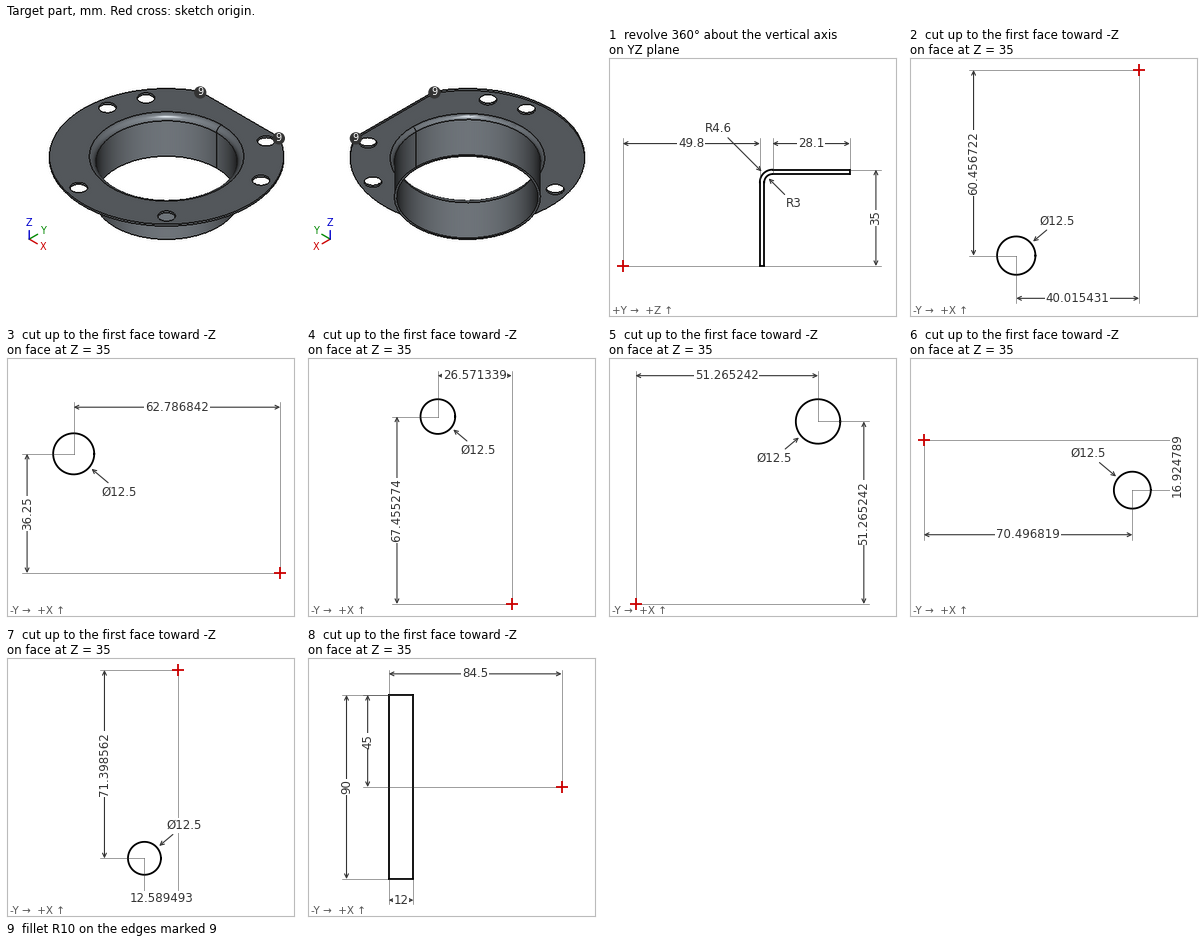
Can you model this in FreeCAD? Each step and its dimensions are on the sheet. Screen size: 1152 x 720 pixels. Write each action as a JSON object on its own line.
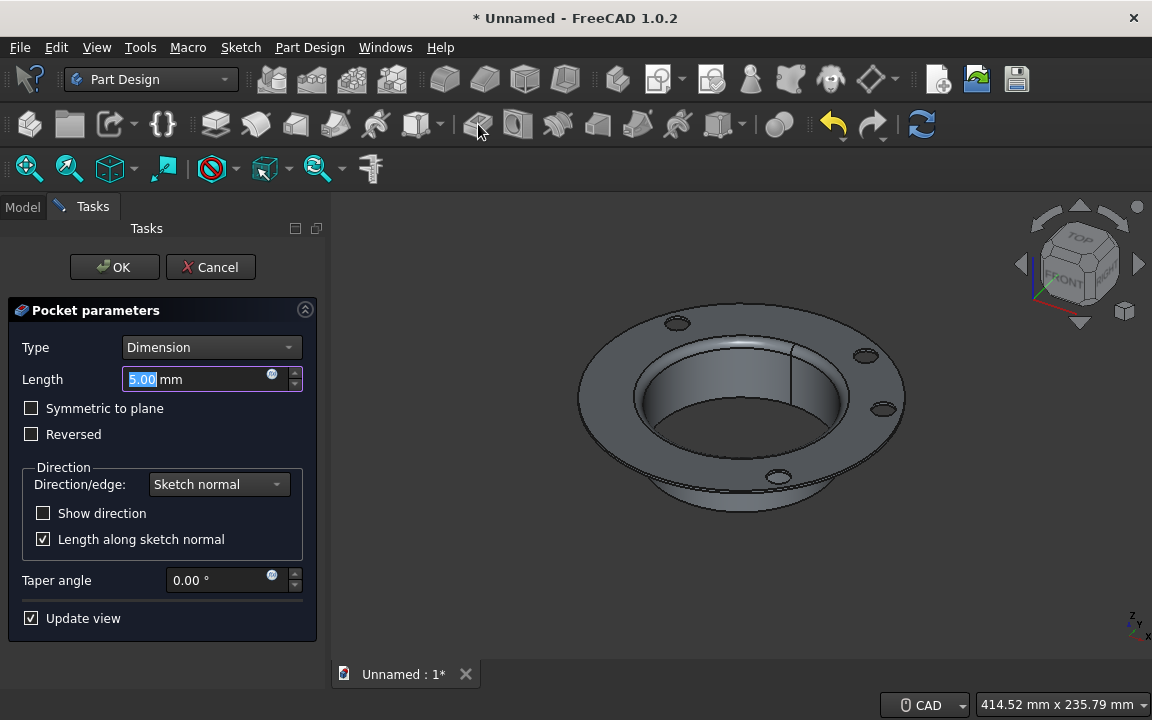
{"action": "left_click", "coordinate": [212, 348]}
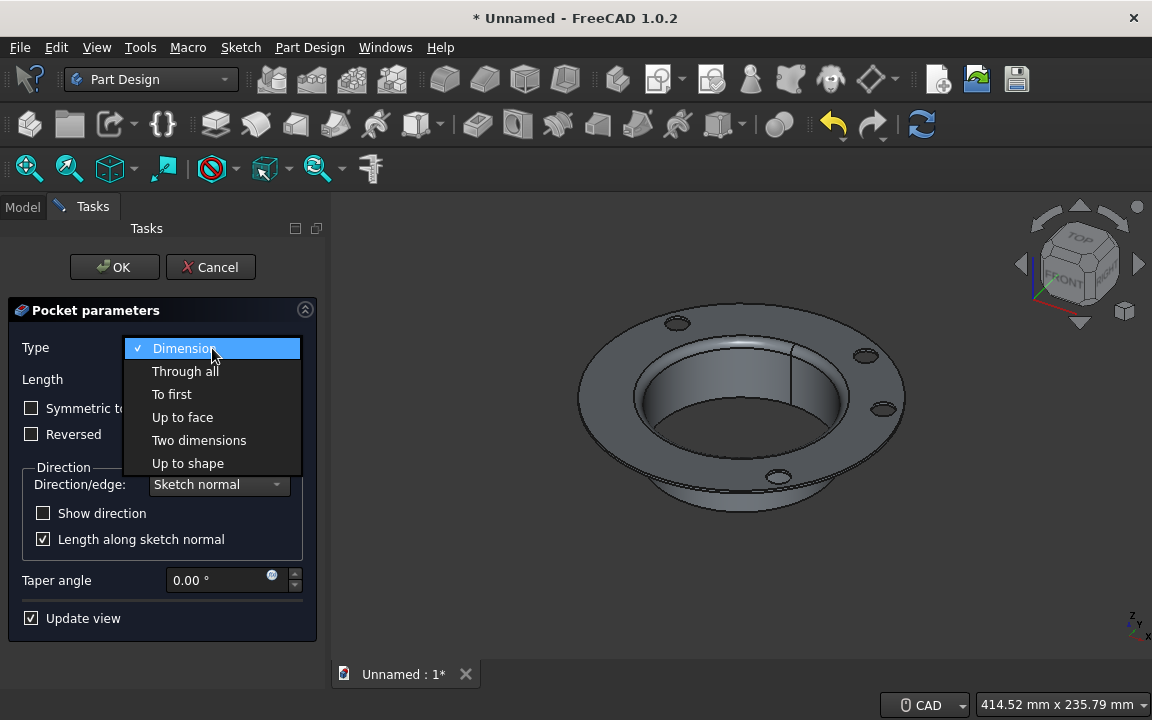
{"action": "left_click", "coordinate": [212, 394]}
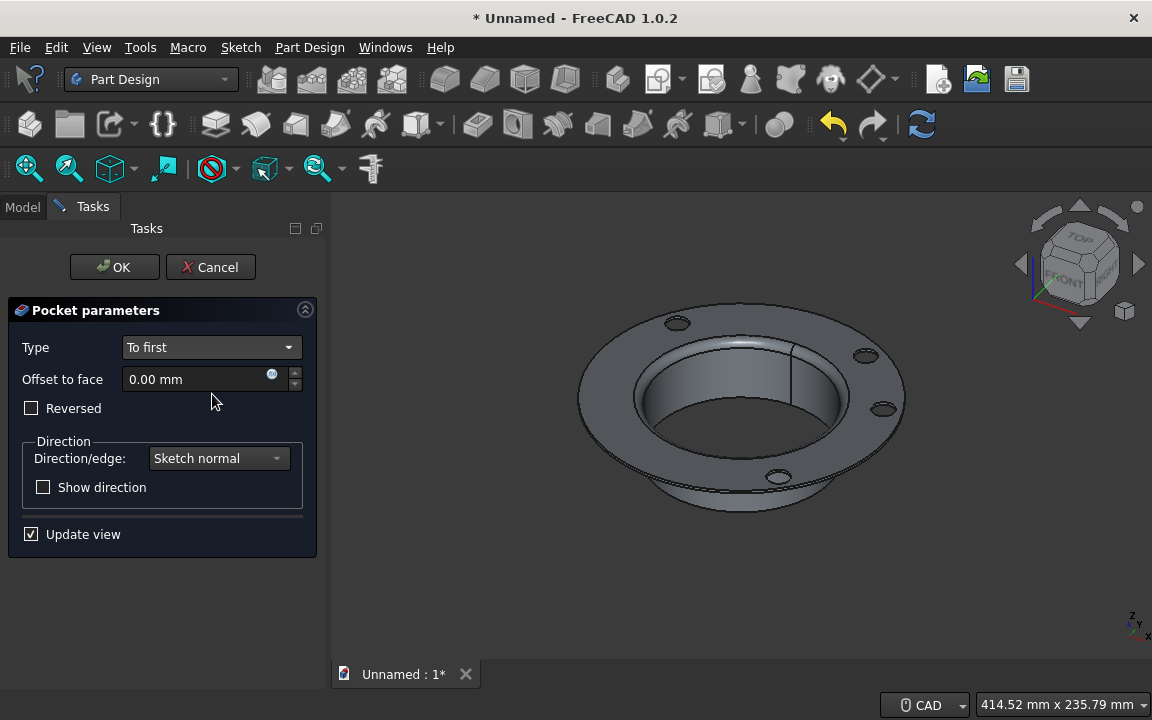
{"action": "left_click", "coordinate": [115, 267]}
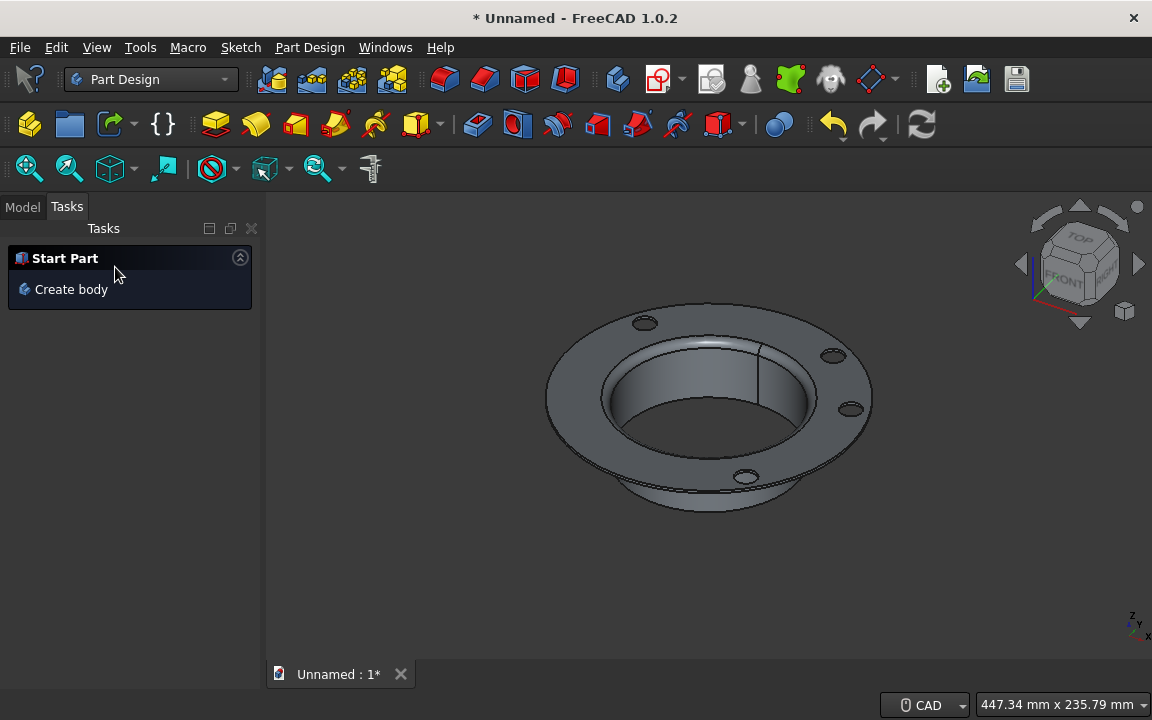
{"action": "left_click", "coordinate": [837, 377]}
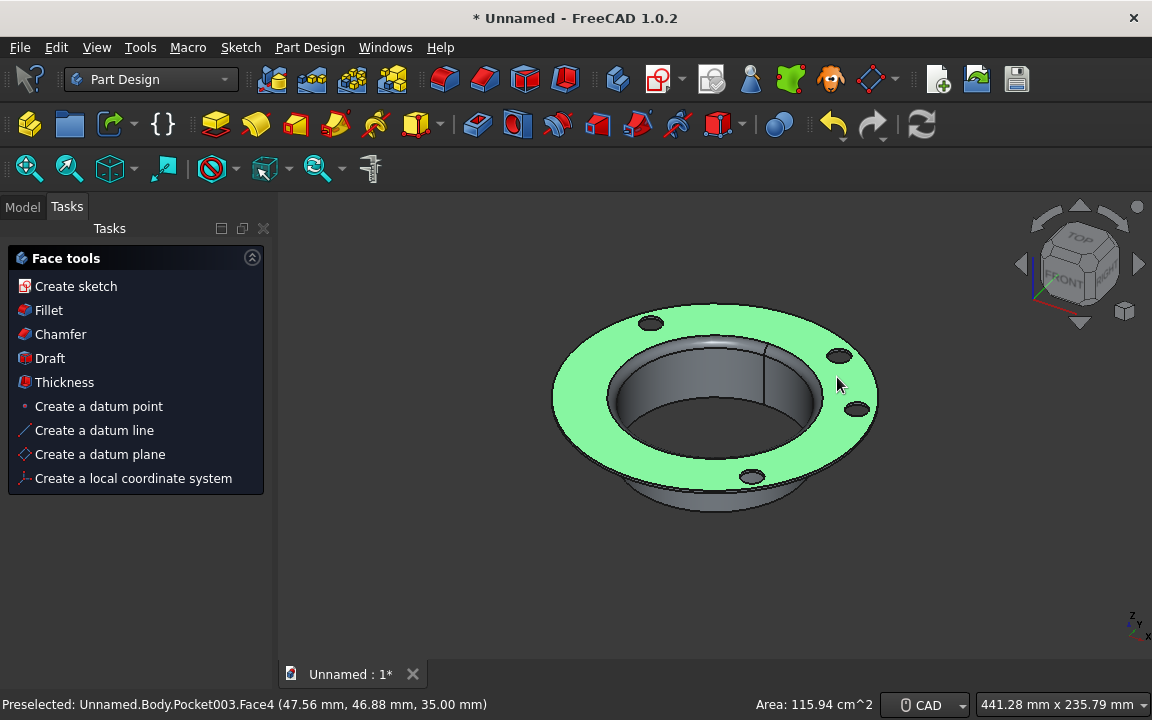
{"action": "left_click", "coordinate": [658, 80]}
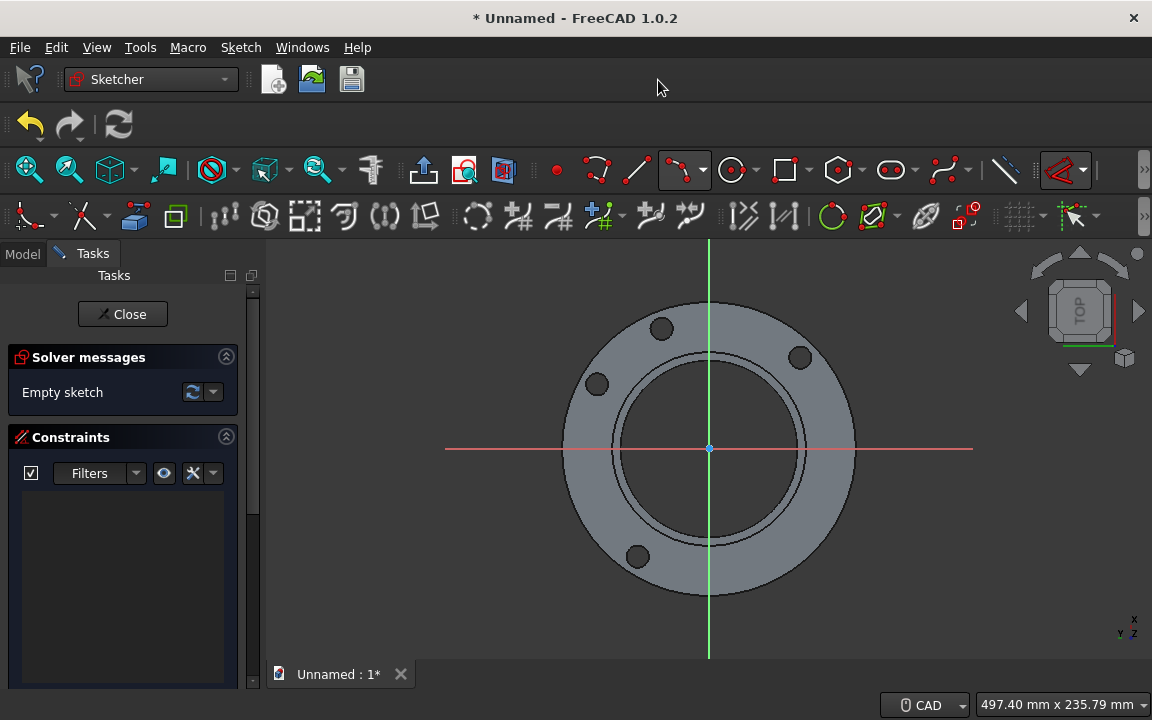
{"action": "scroll", "coordinate": [854, 482], "scroll_direction": "up", "scroll_amount": 12}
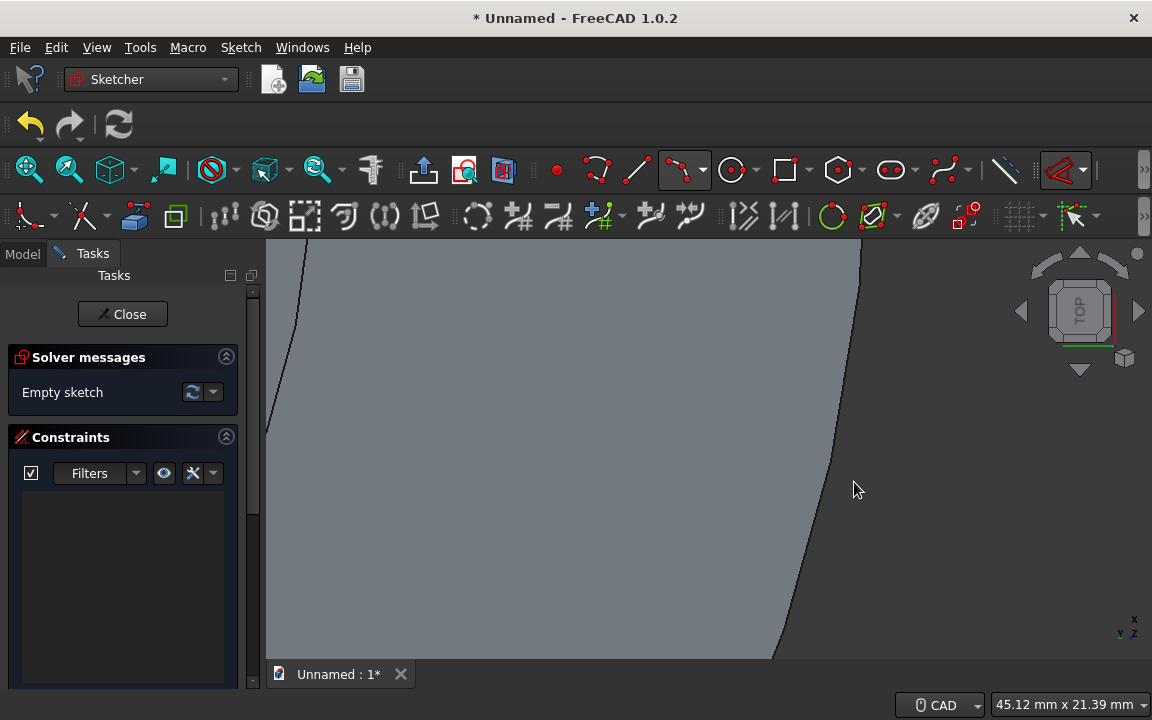
{"action": "key", "text": "g c"}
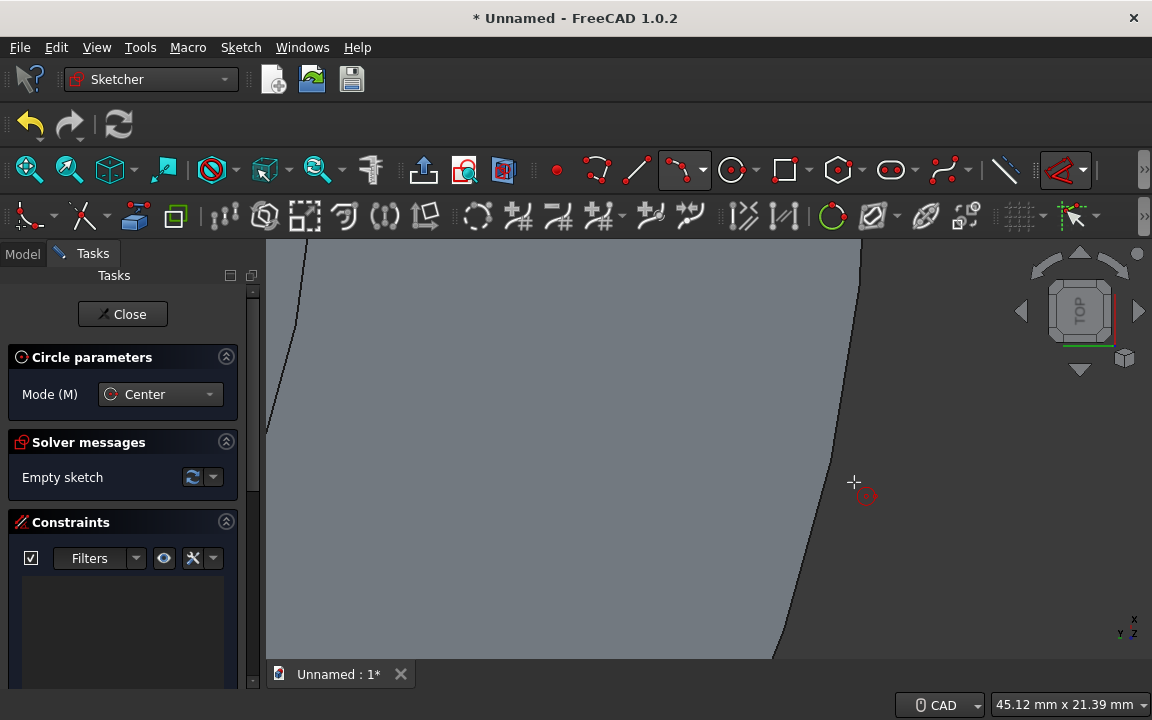
{"action": "left_click", "coordinate": [633, 445]}
{"action": "mouse_move", "coordinate": [720, 358]}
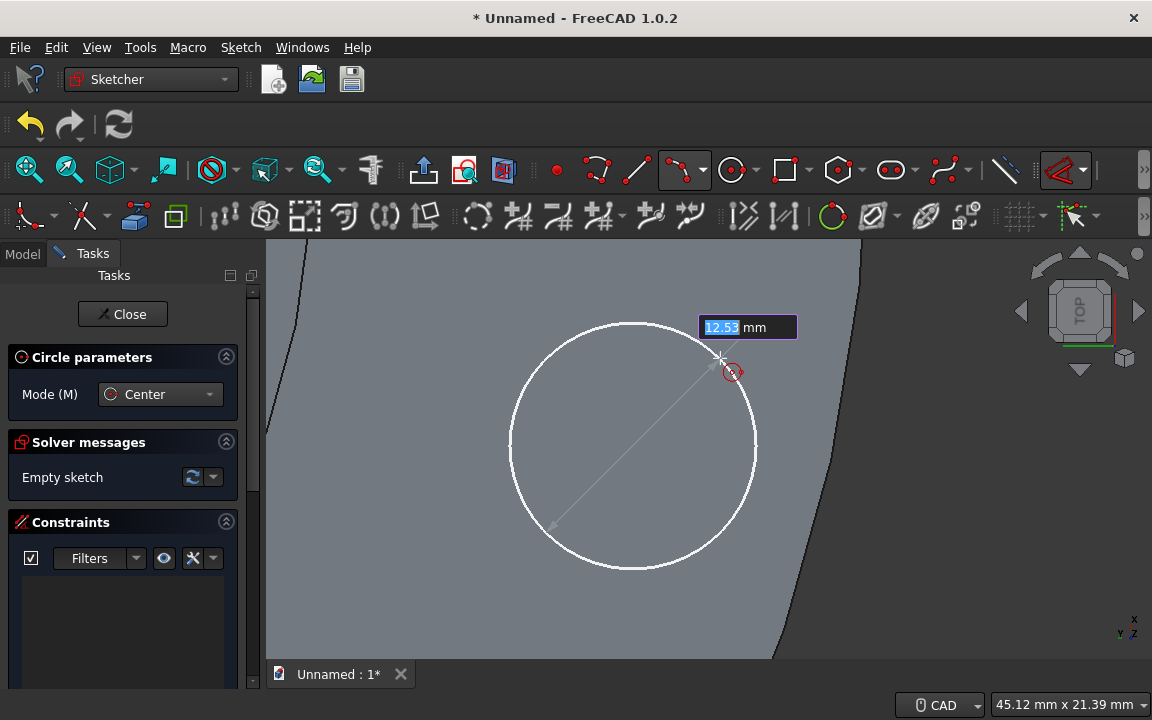
{"action": "type", "text": "12.5"}
{"action": "key", "text": "Return"}
{"action": "key", "text": "Escape"}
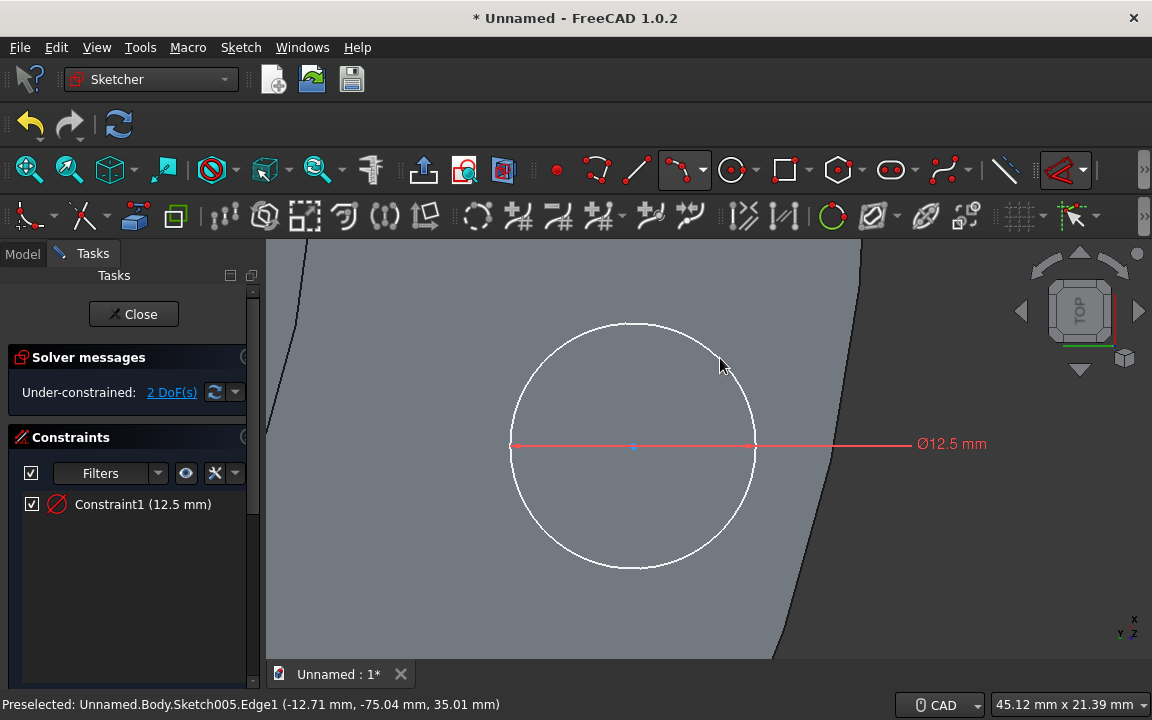
{"action": "left_click", "coordinate": [633, 446]}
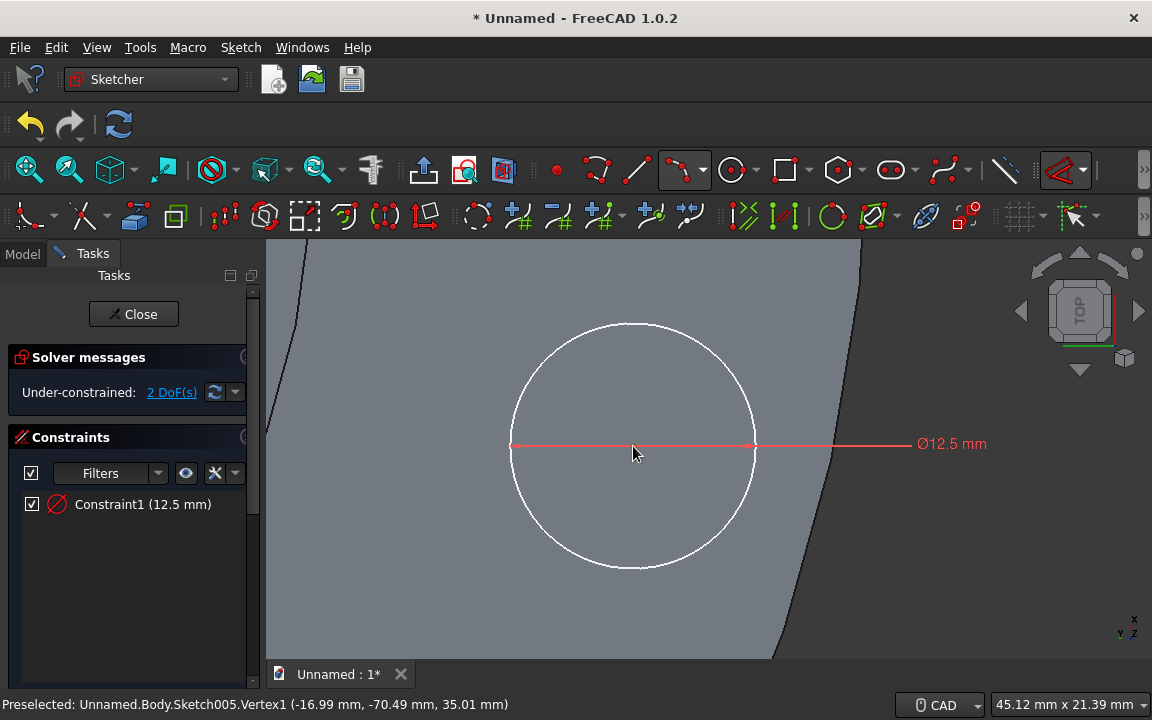
{"action": "key", "text": "l"}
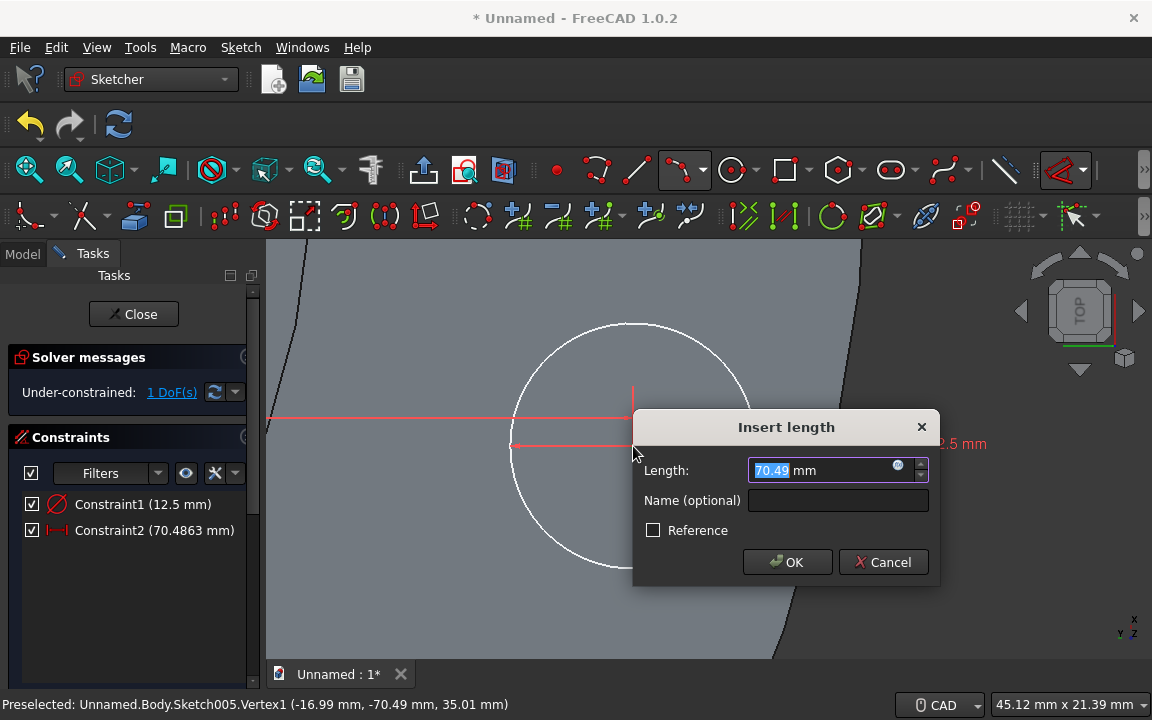
{"action": "type", "text": "70.496819"}
{"action": "key", "text": "Return"}